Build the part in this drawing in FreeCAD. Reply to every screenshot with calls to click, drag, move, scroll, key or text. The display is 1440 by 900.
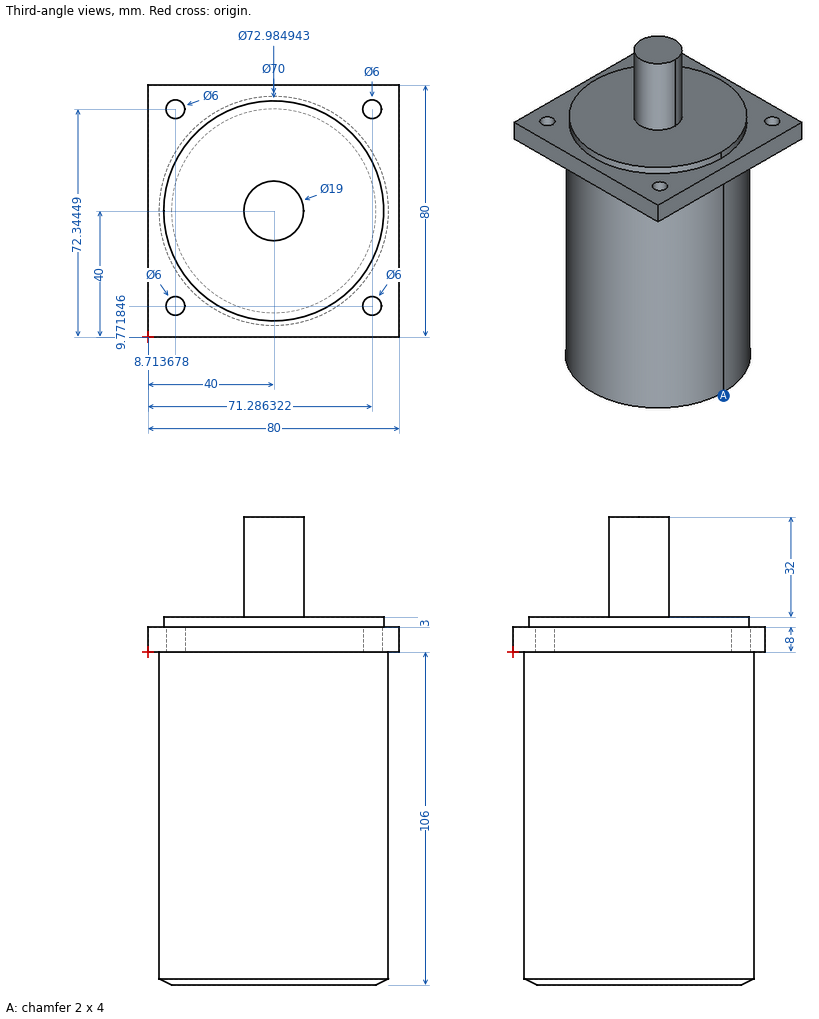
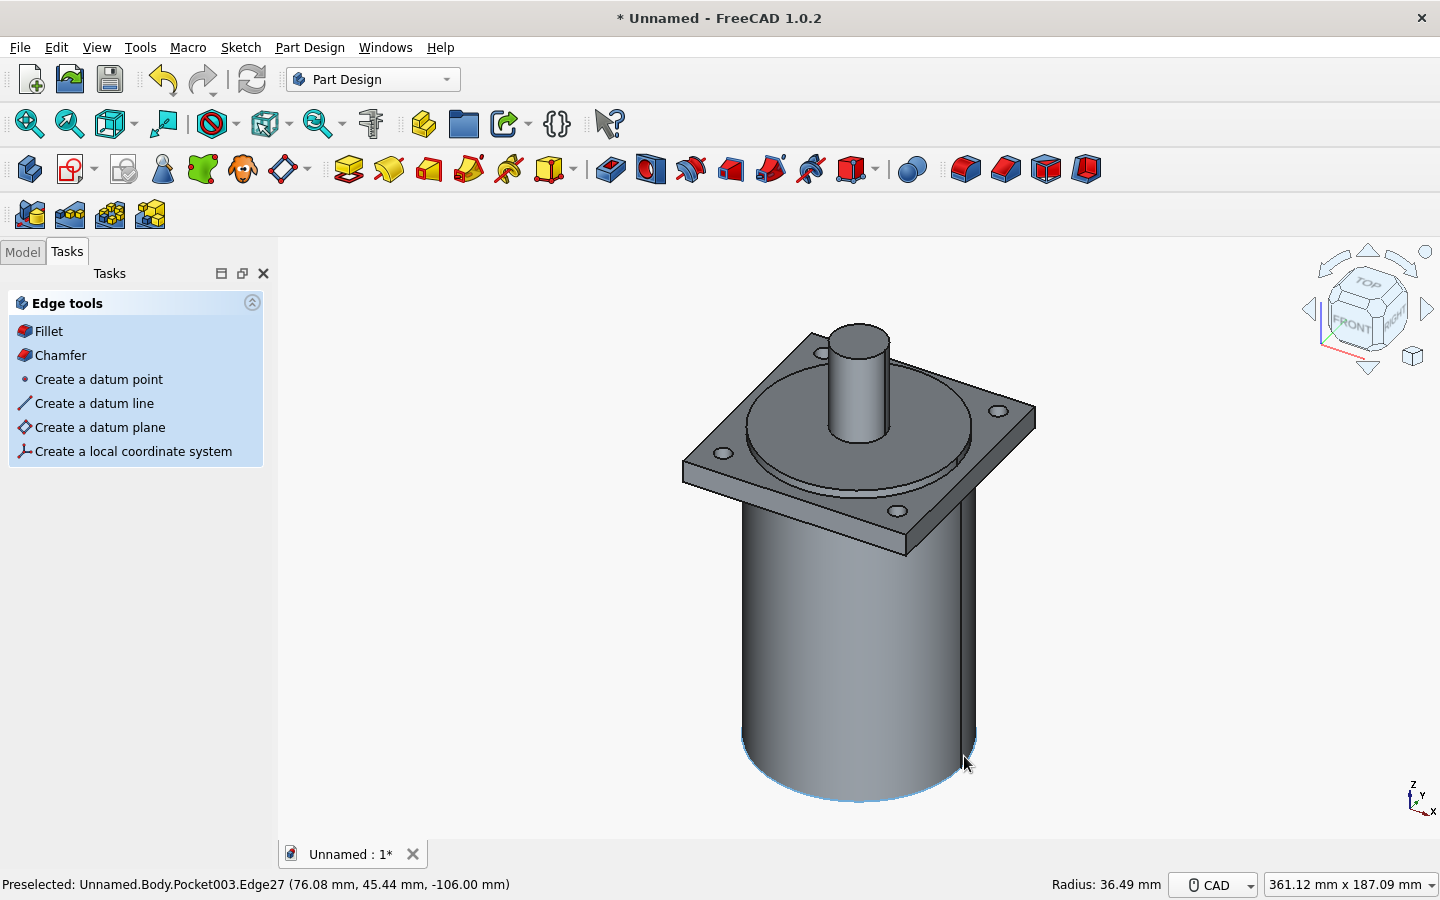
click(1006, 170)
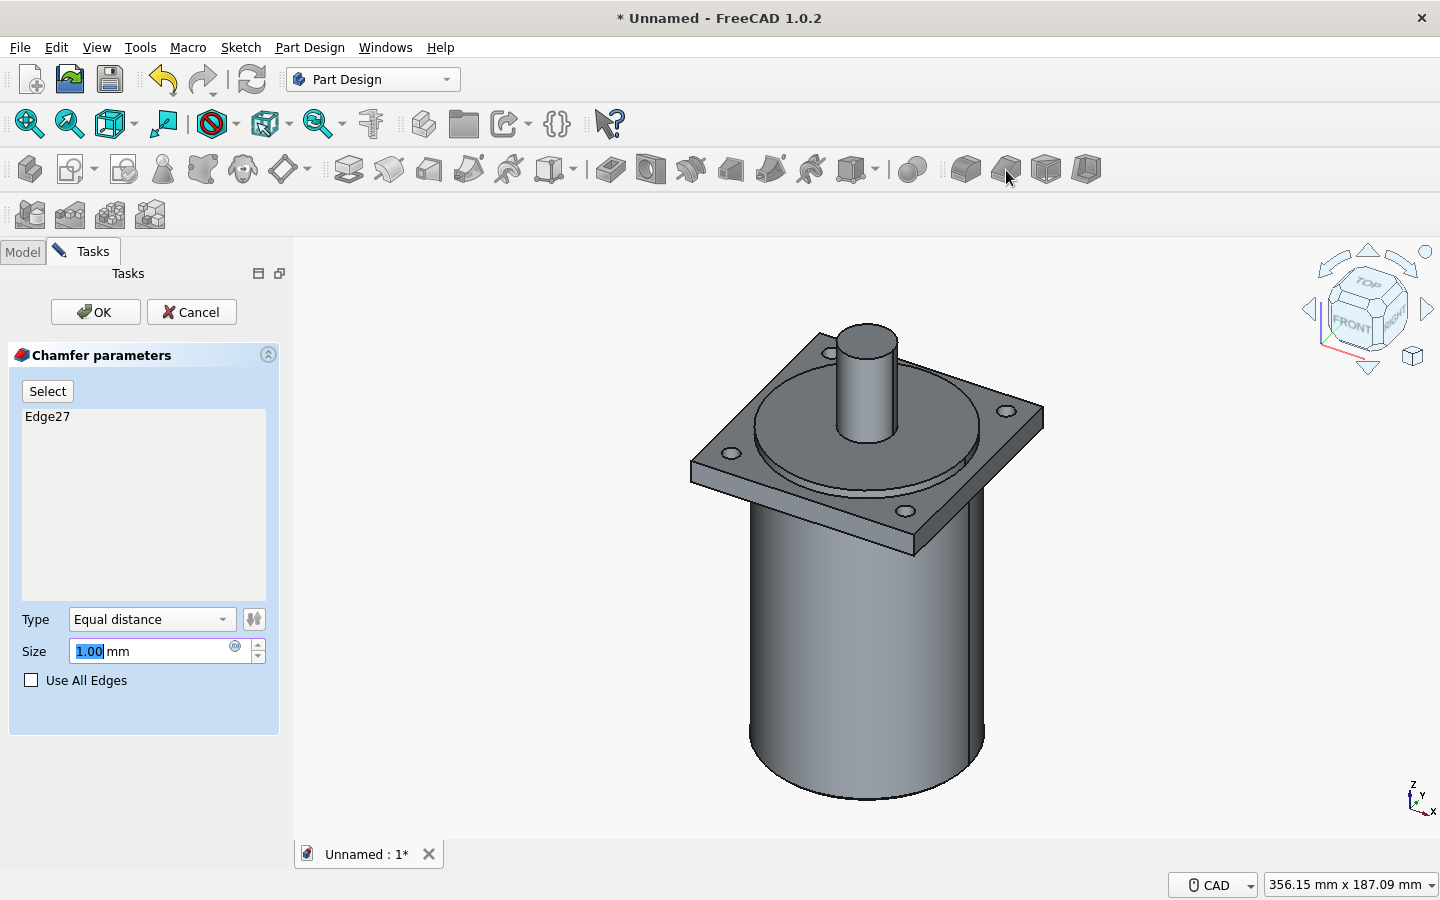
text(2)
key(Tab)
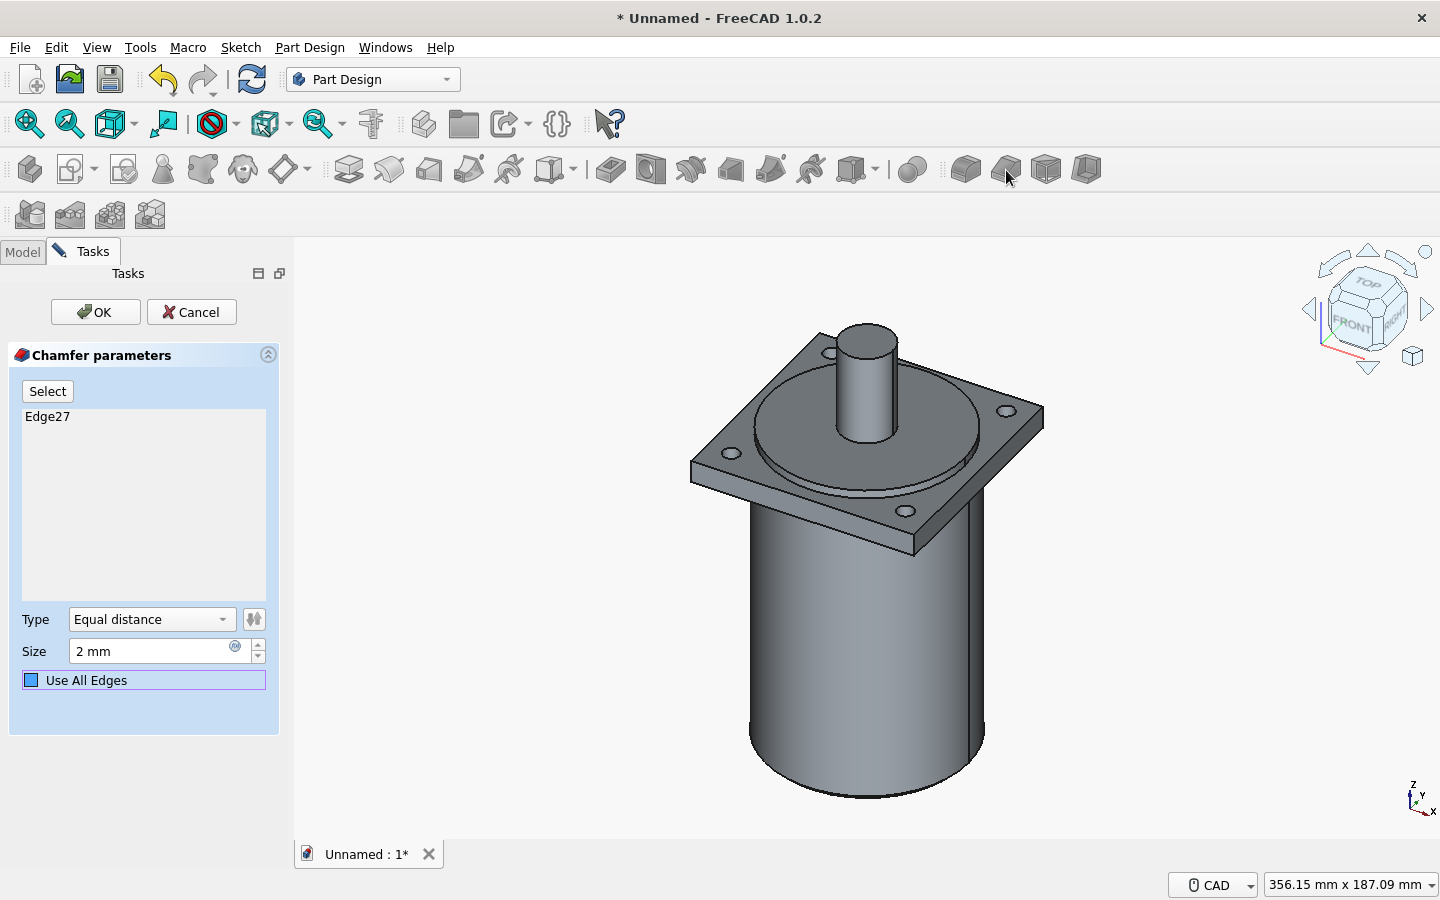
click(153, 620)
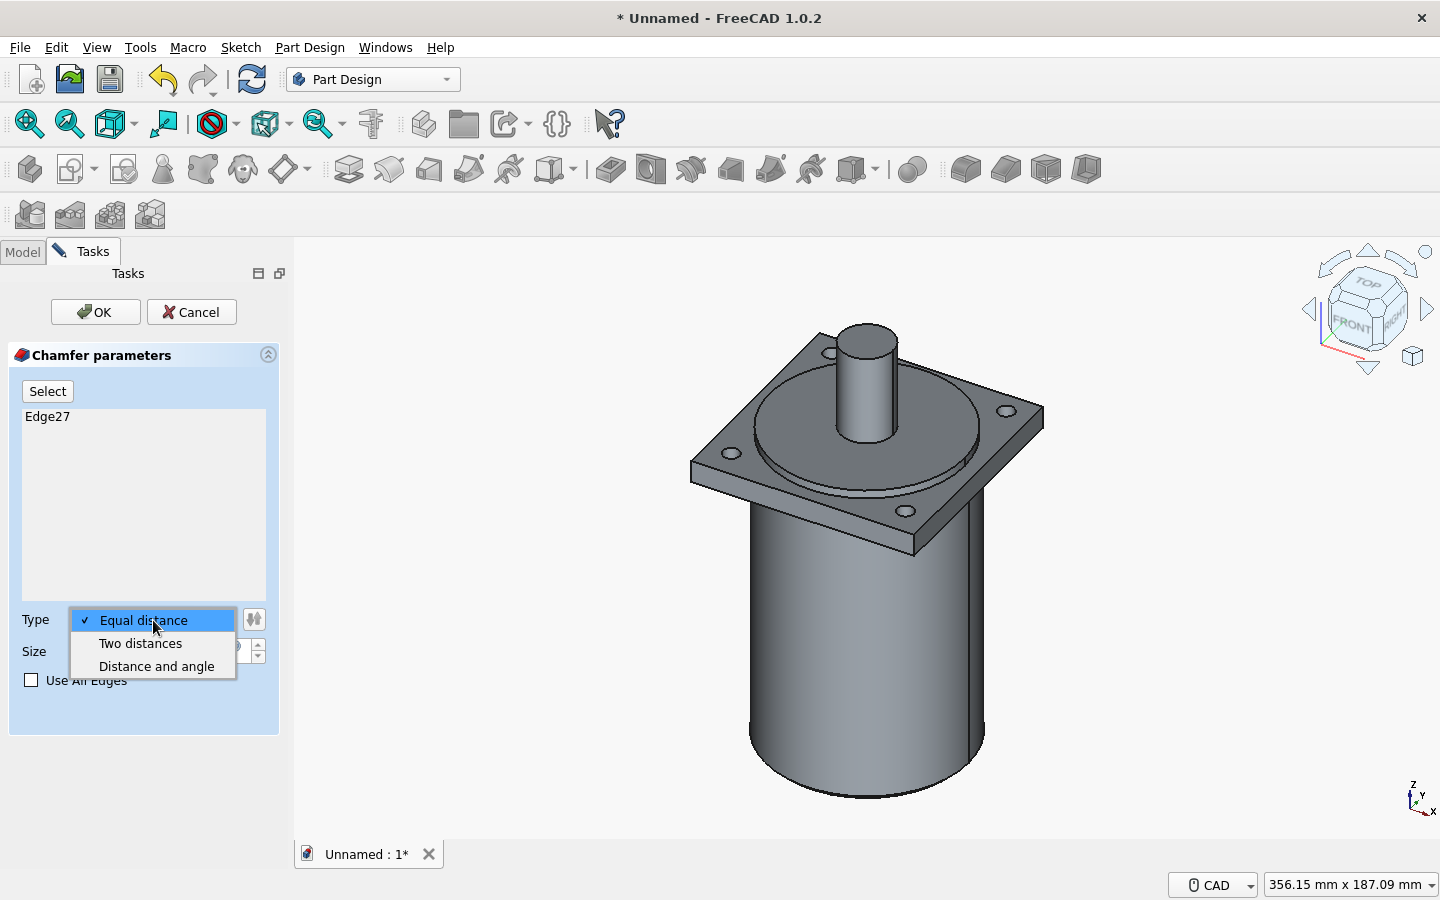
click(152, 644)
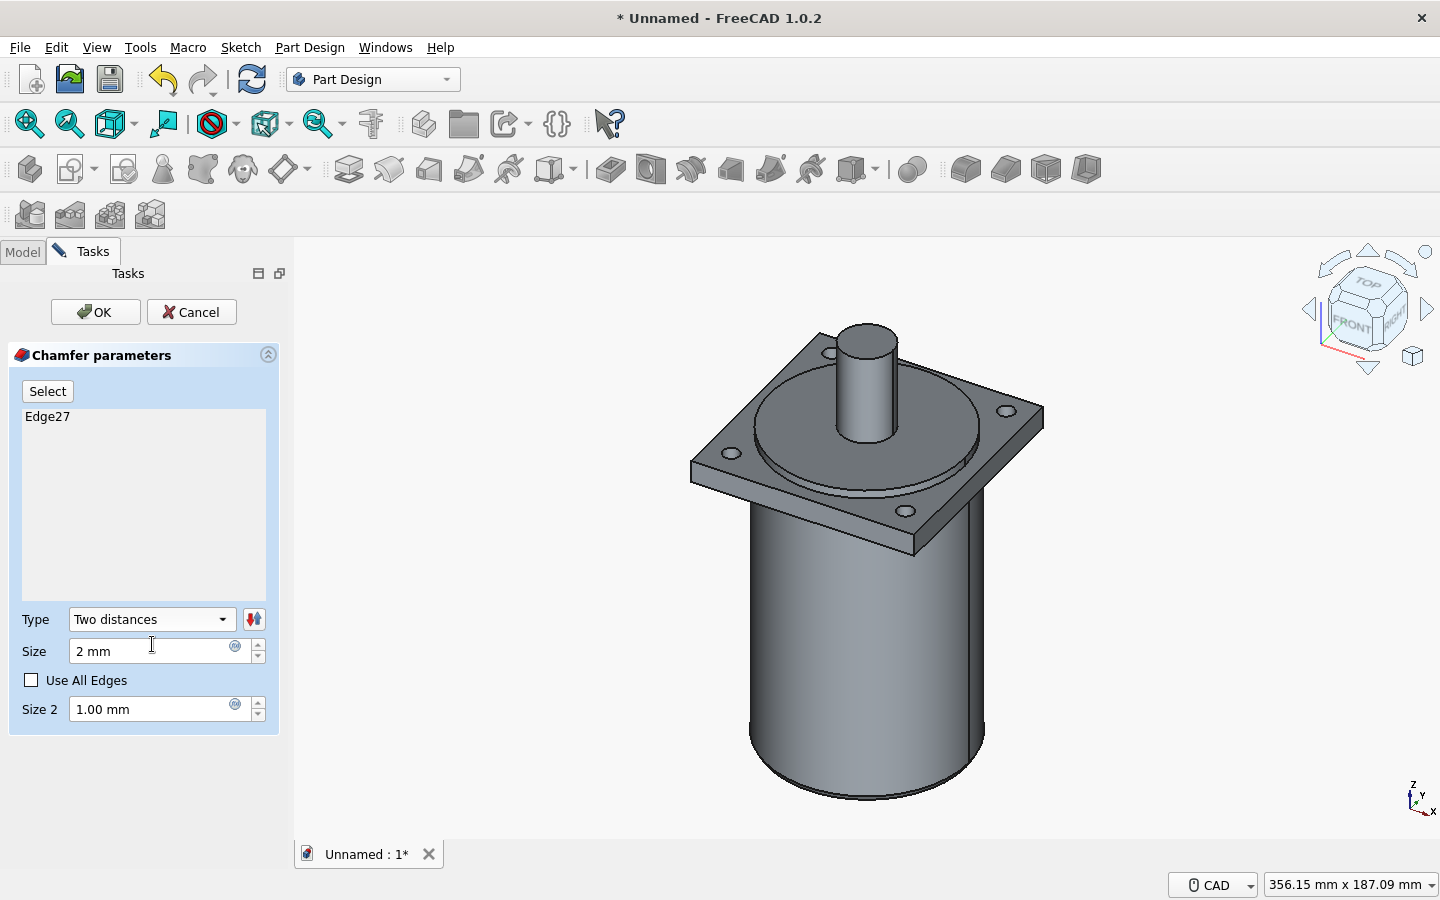
triple_click(160, 709)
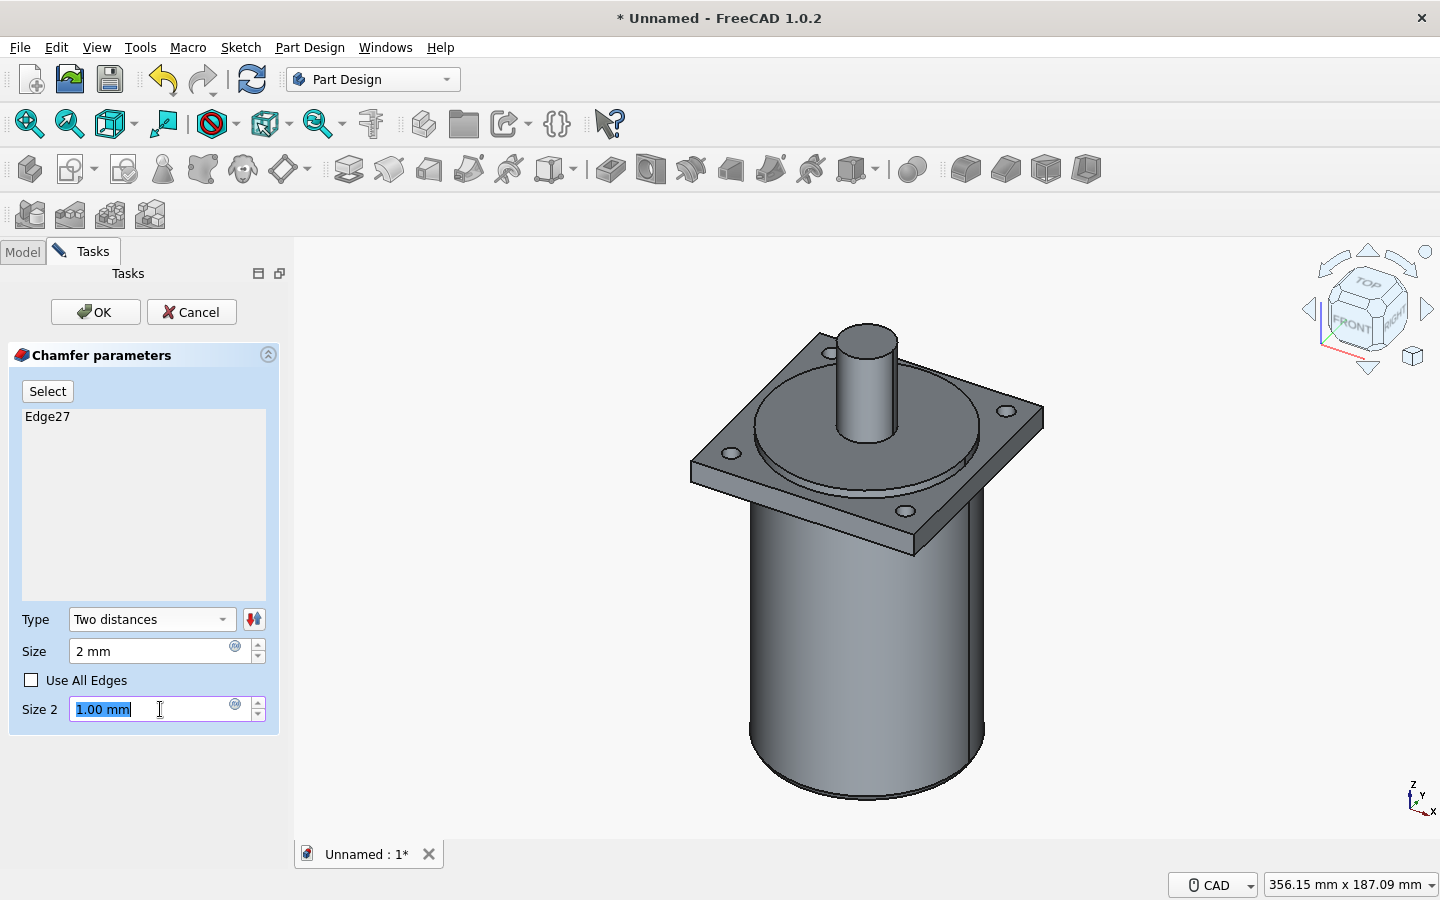
text(4)
key(Tab)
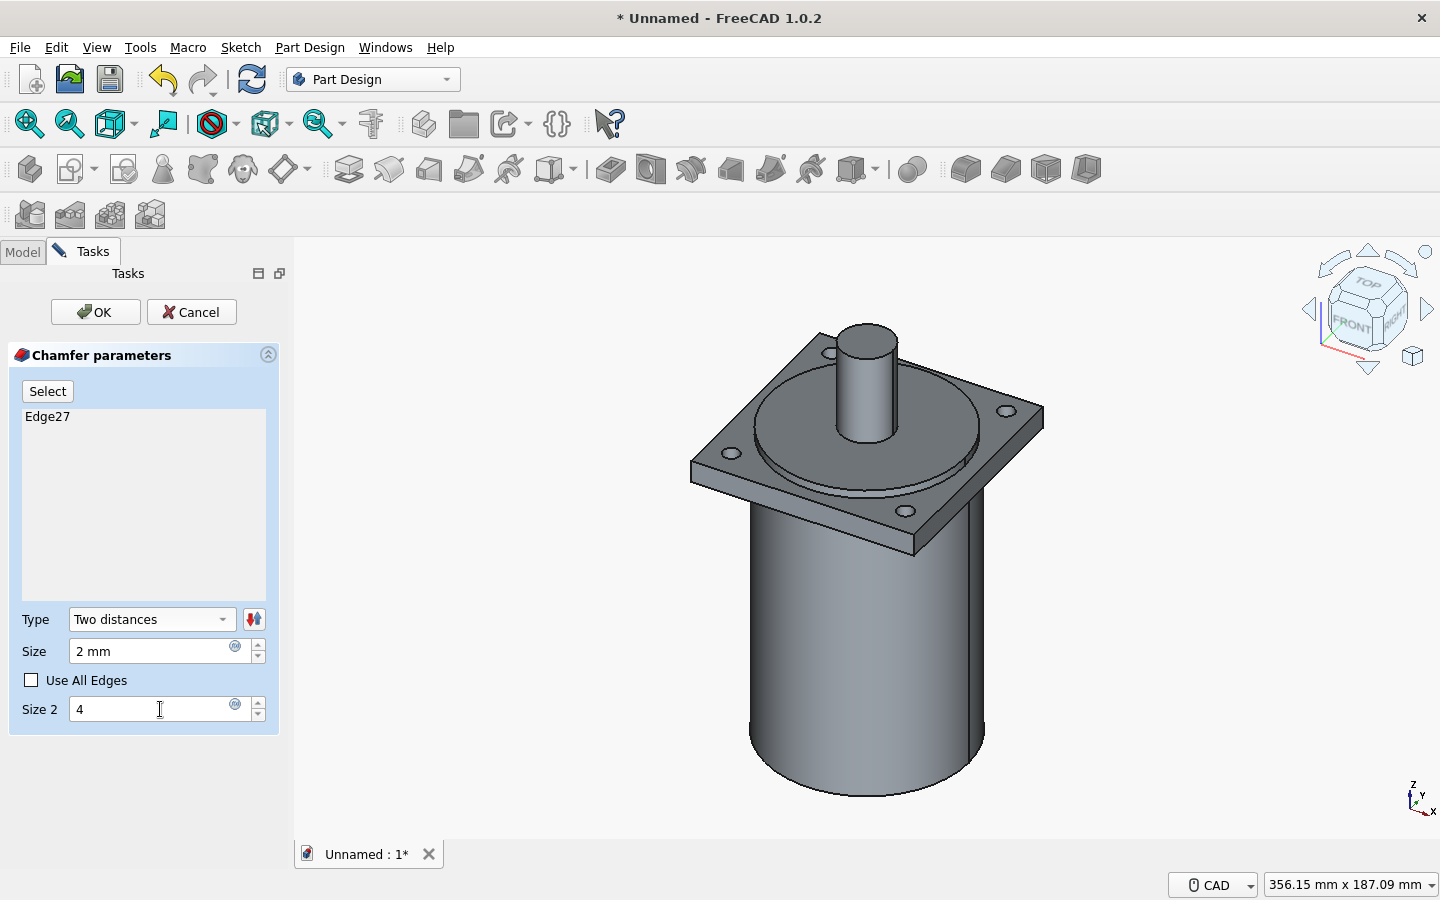
click(96, 312)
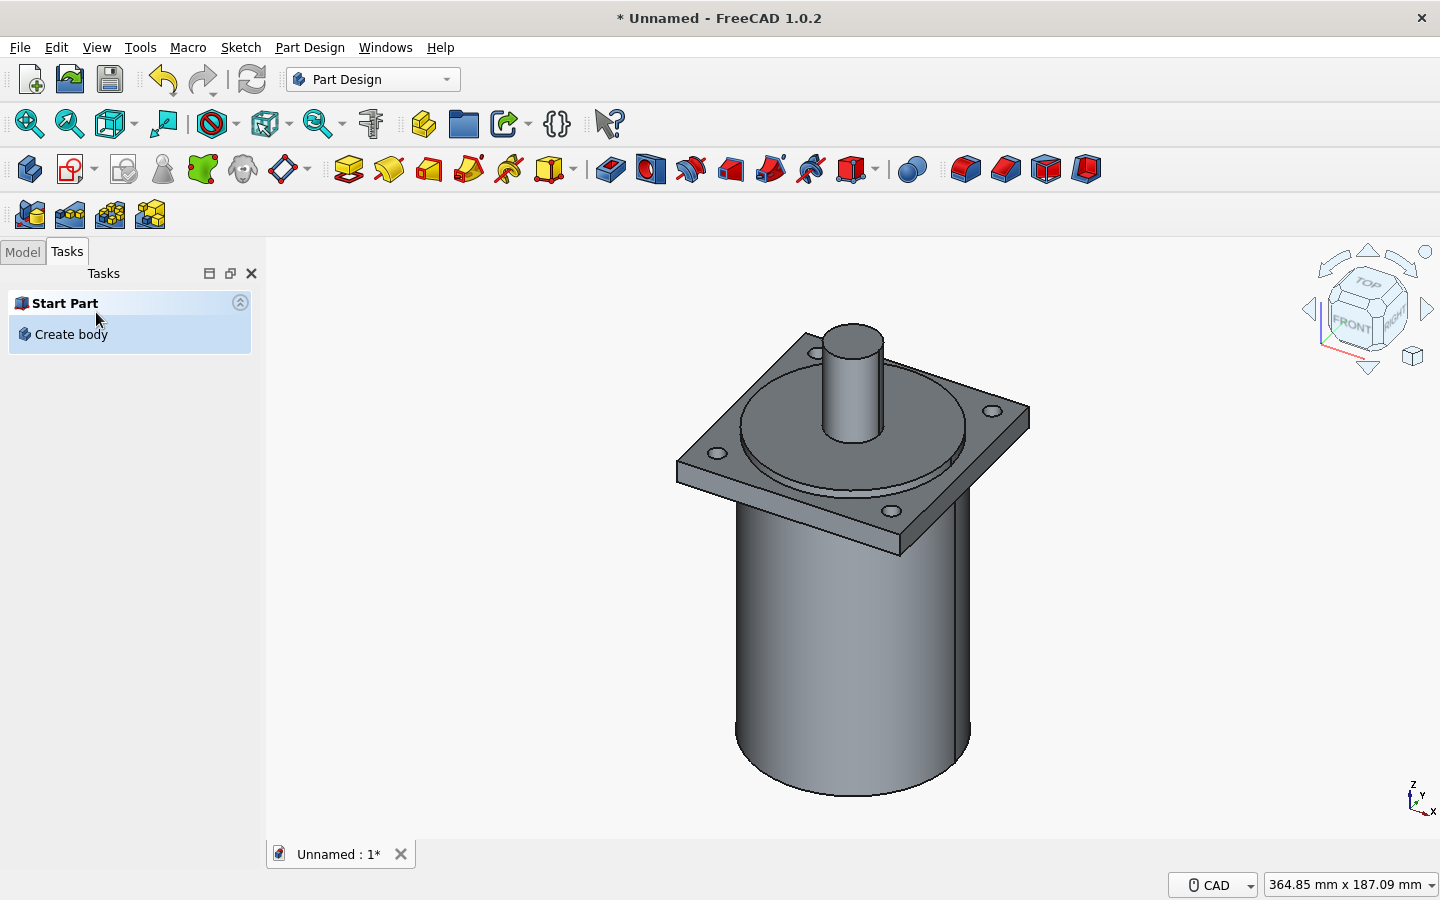
key(0)